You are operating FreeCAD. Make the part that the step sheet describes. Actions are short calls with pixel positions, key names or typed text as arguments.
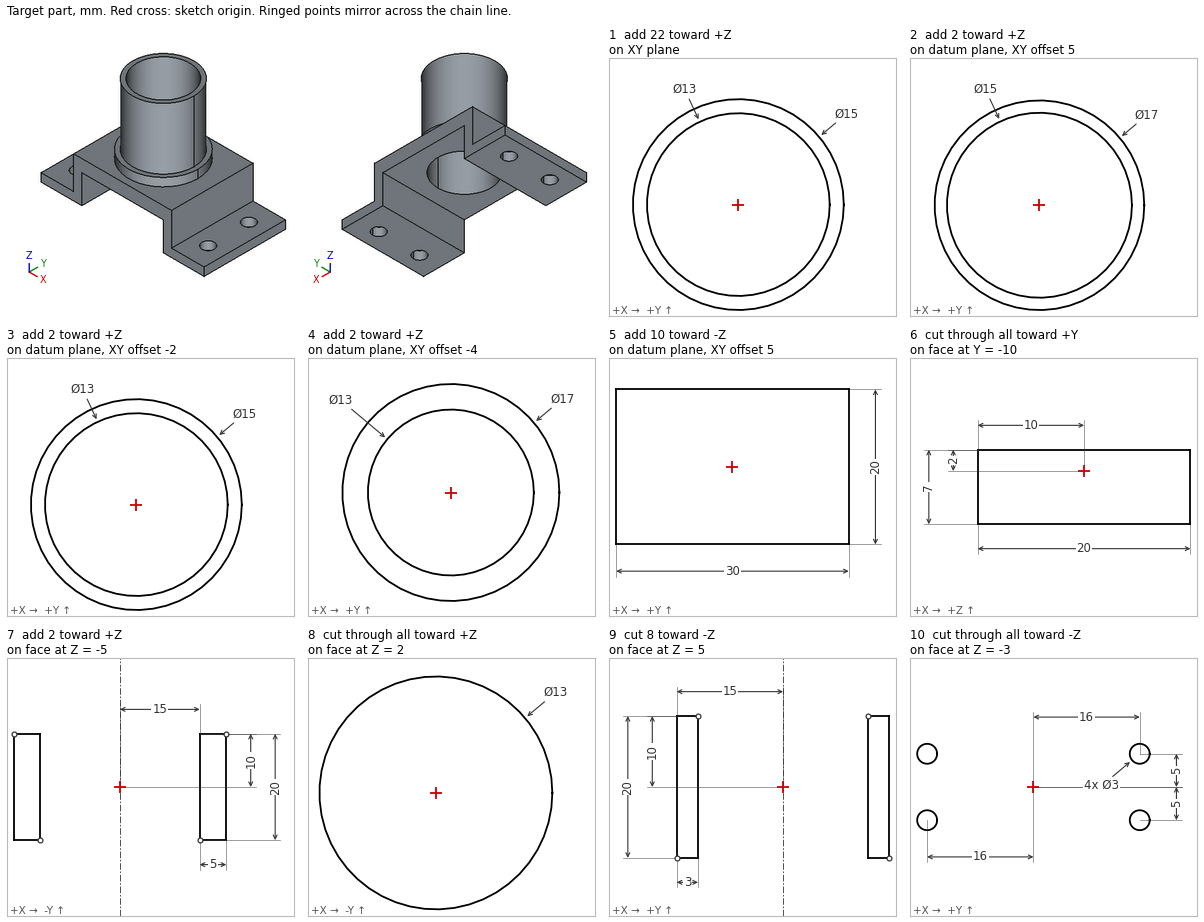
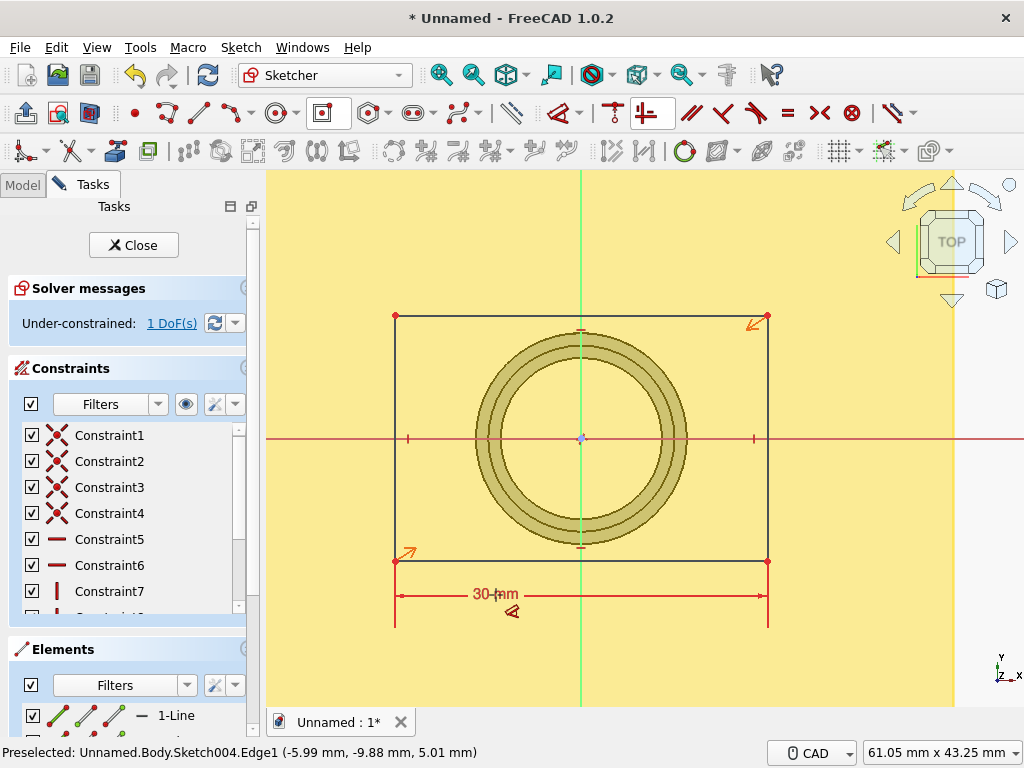
click(768, 488)
click(802, 382)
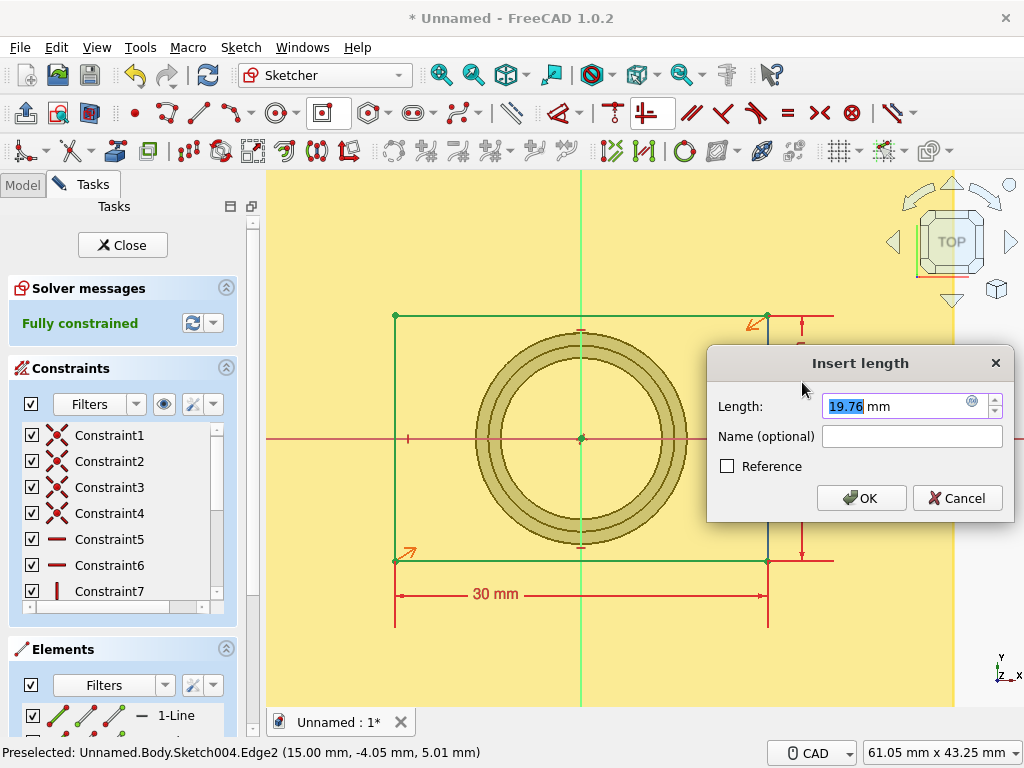
text(20)
key(Return)
key(Escape)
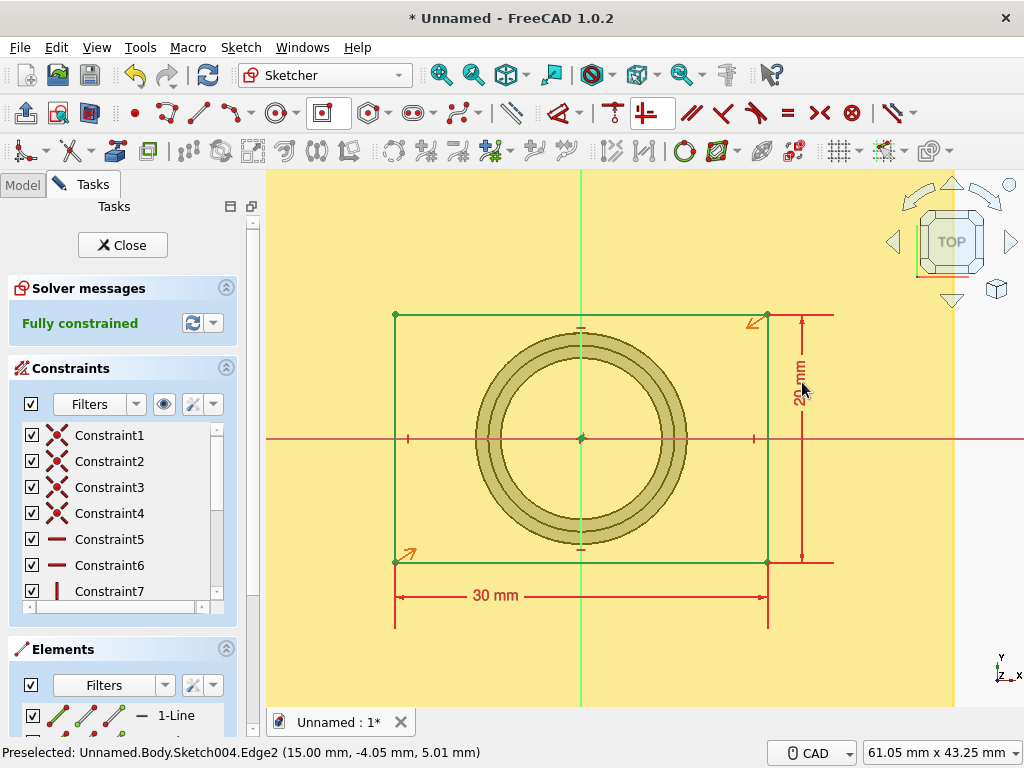
click(123, 245)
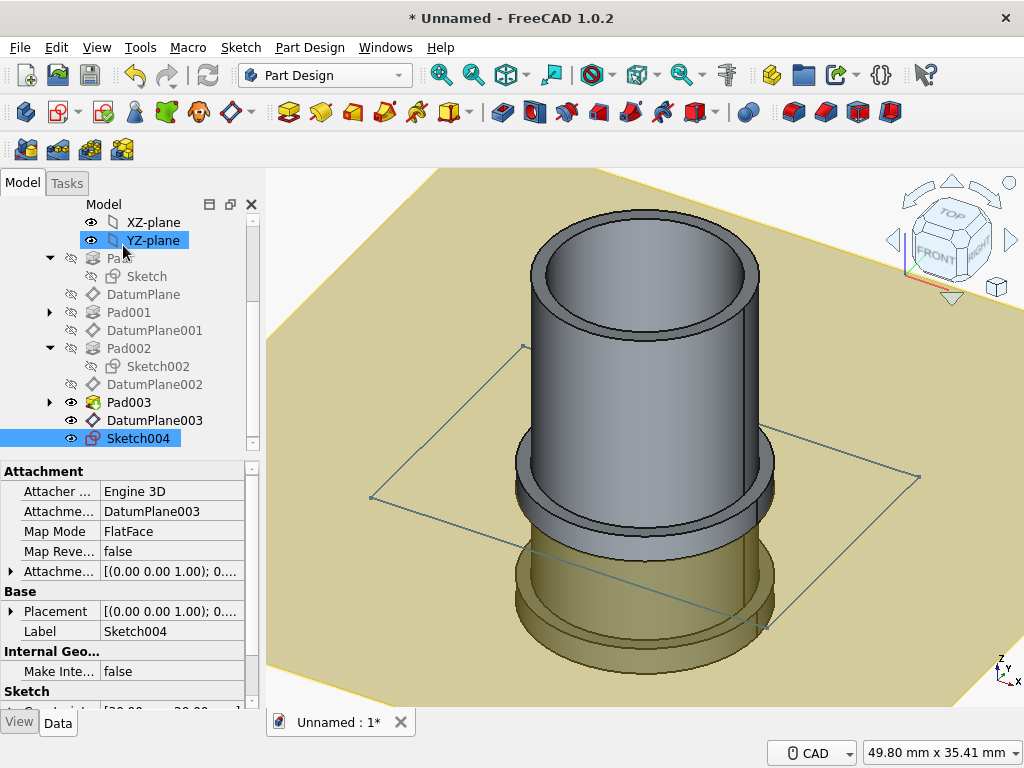
click(290, 112)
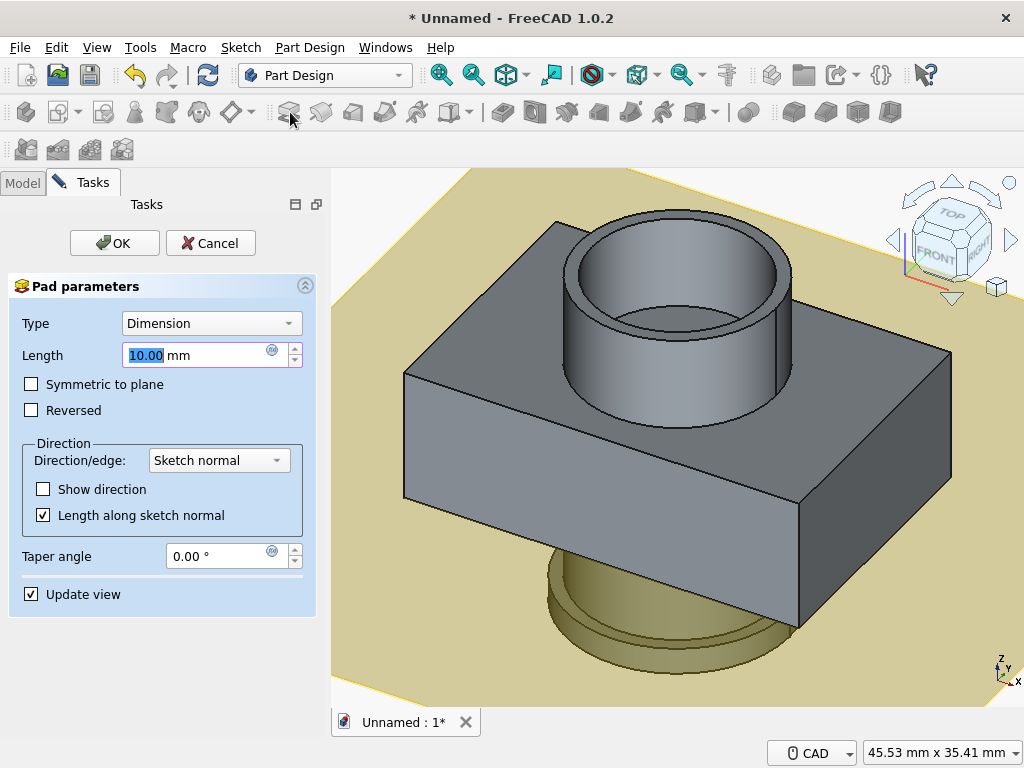
text(10)
key(Tab)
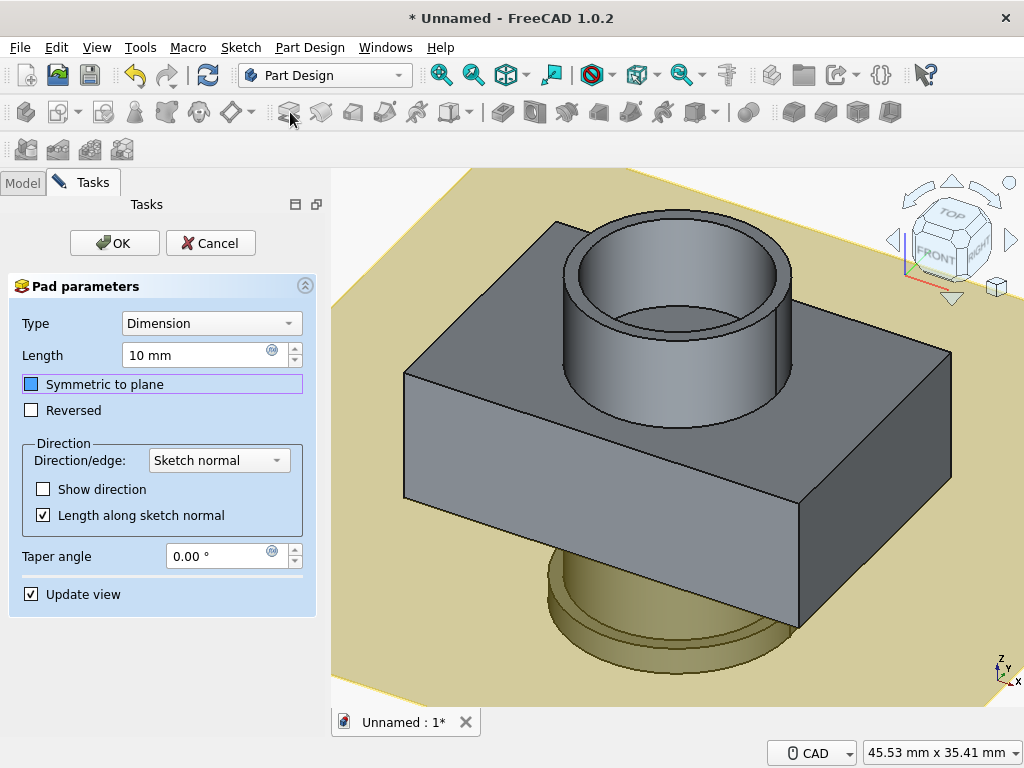
click(30, 410)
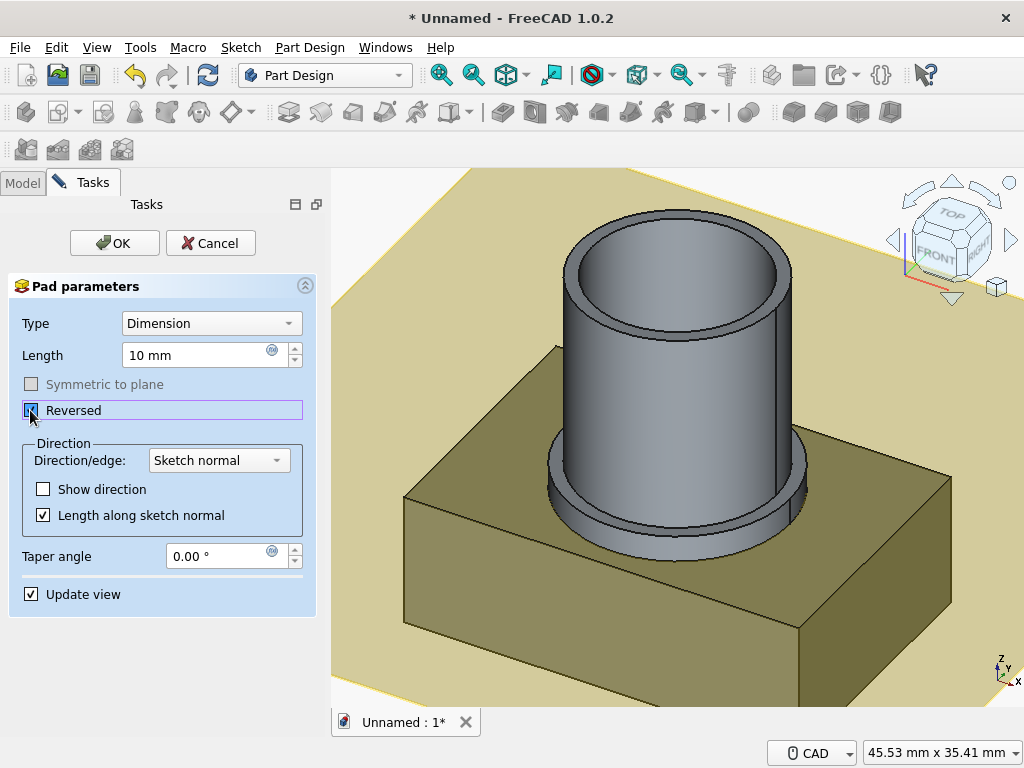
click(115, 243)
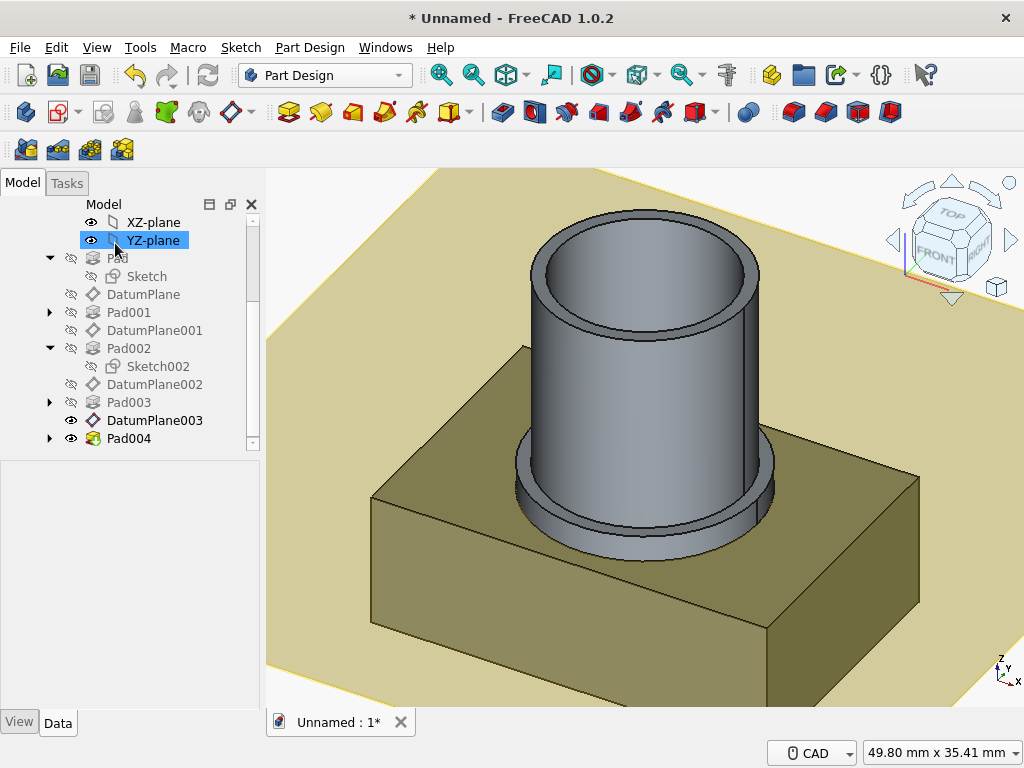
click(116, 420)
key(space)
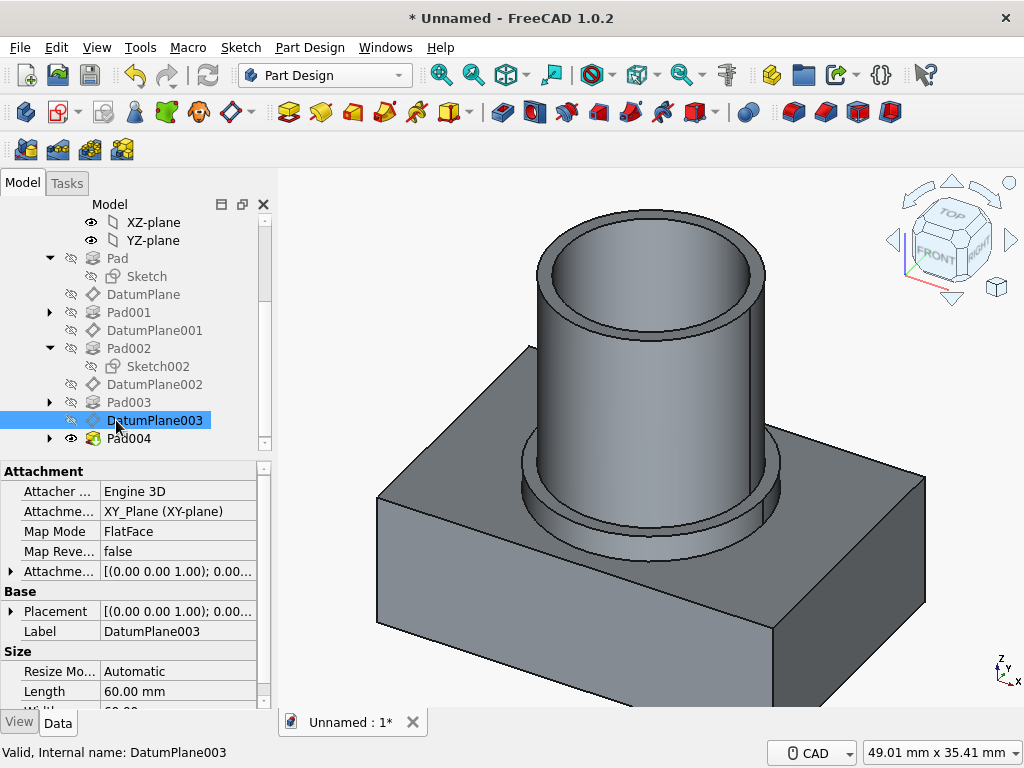
key(v)
key(f)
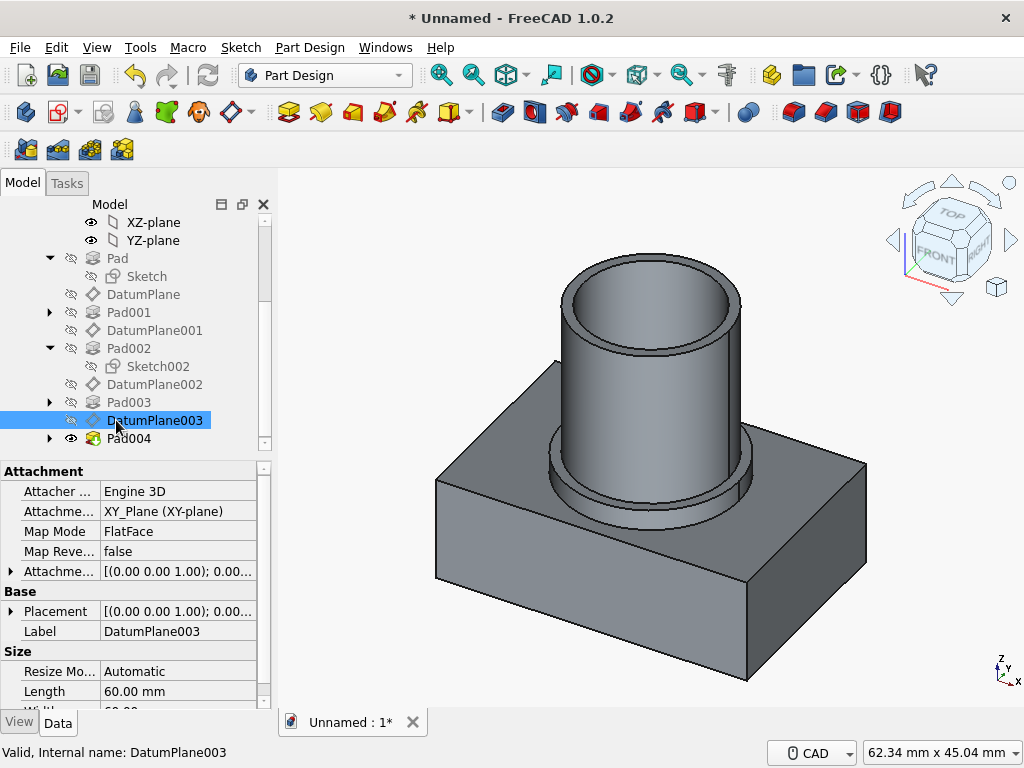
click(680, 609)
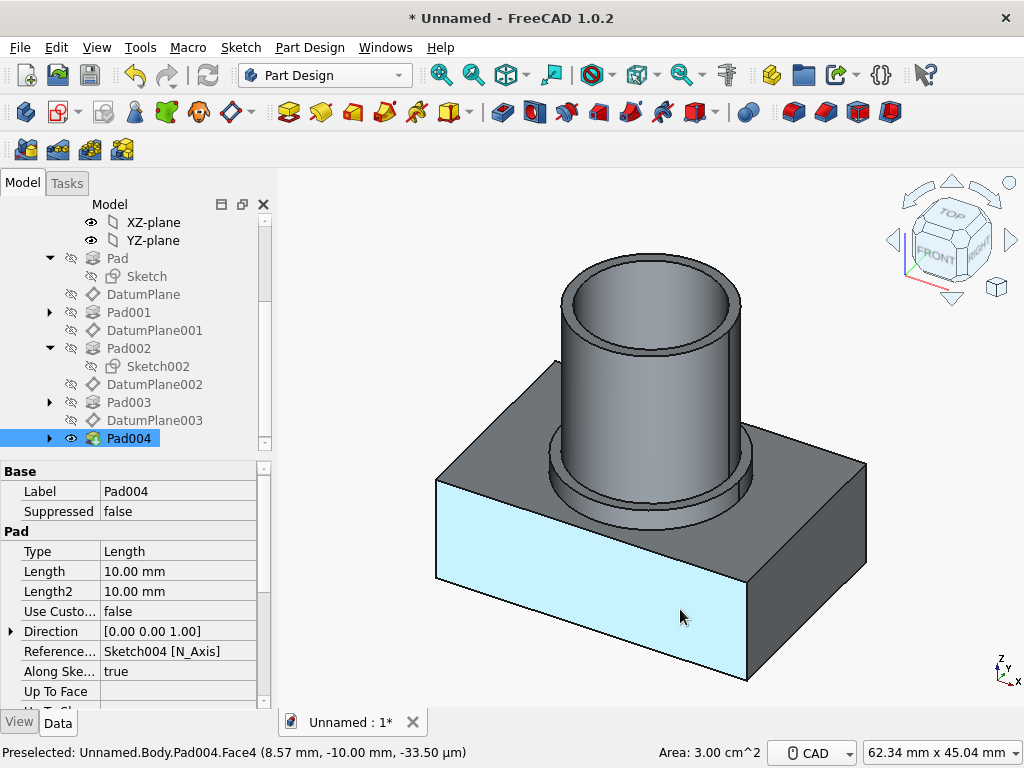
click(58, 112)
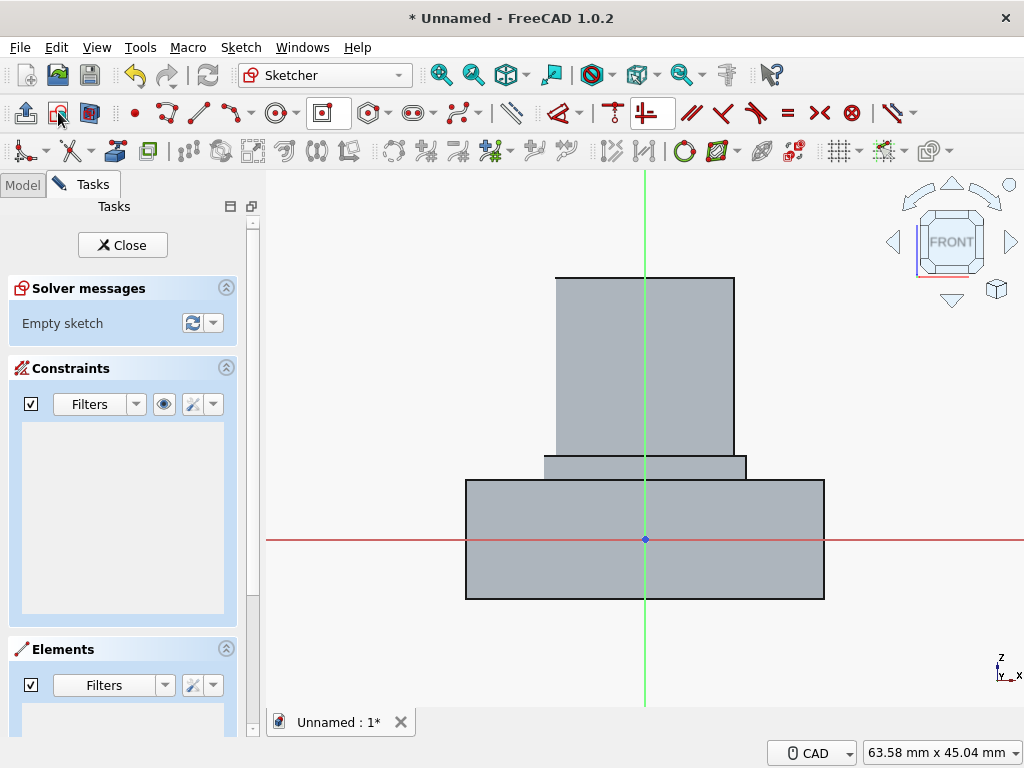
scroll(728, 679, up, 3)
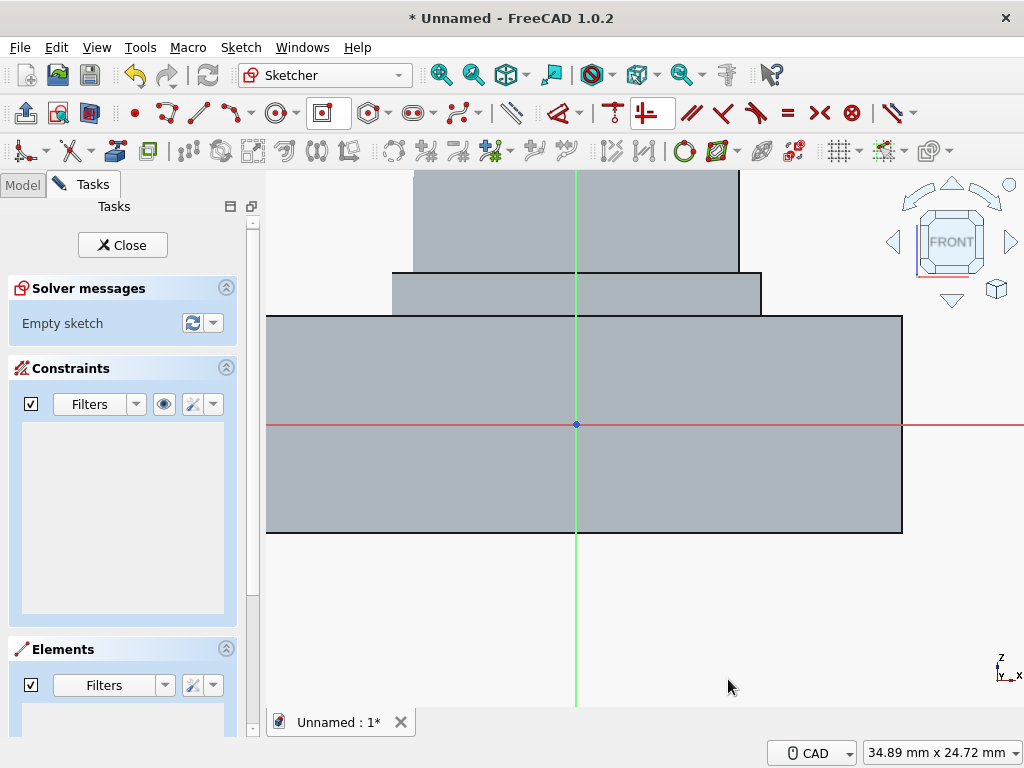
key(g)
key(r)